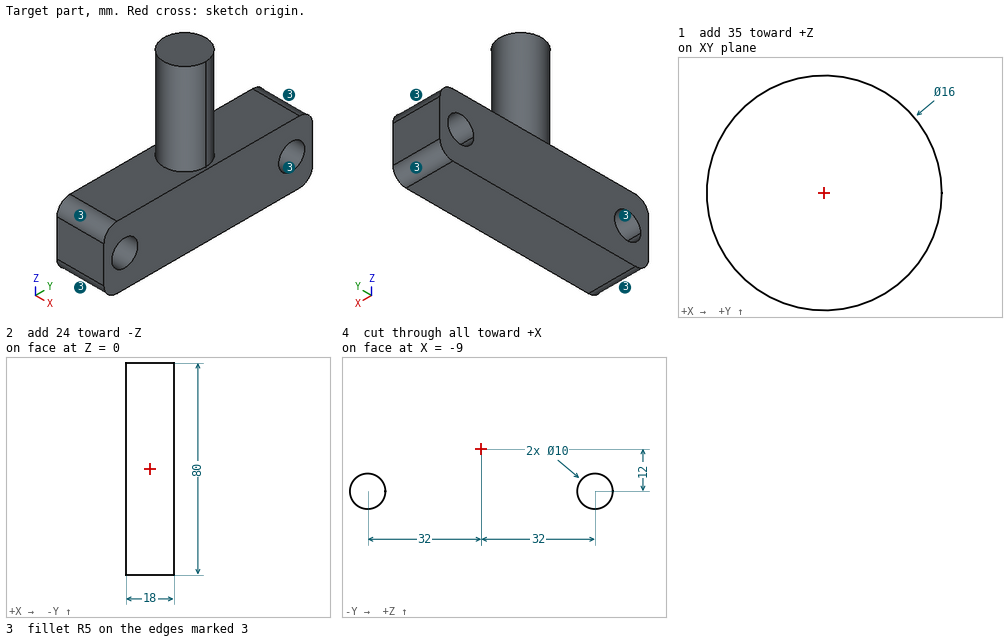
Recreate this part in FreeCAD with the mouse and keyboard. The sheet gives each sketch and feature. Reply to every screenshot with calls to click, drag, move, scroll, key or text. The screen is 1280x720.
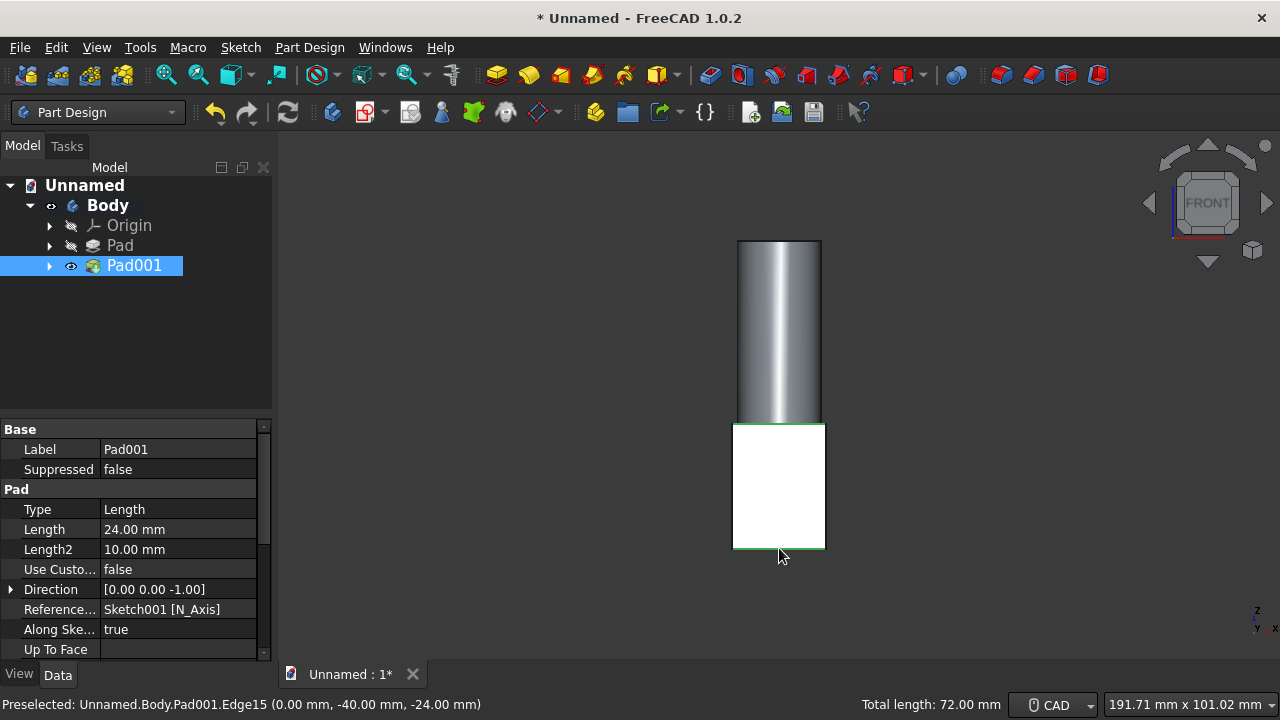
click(1002, 76)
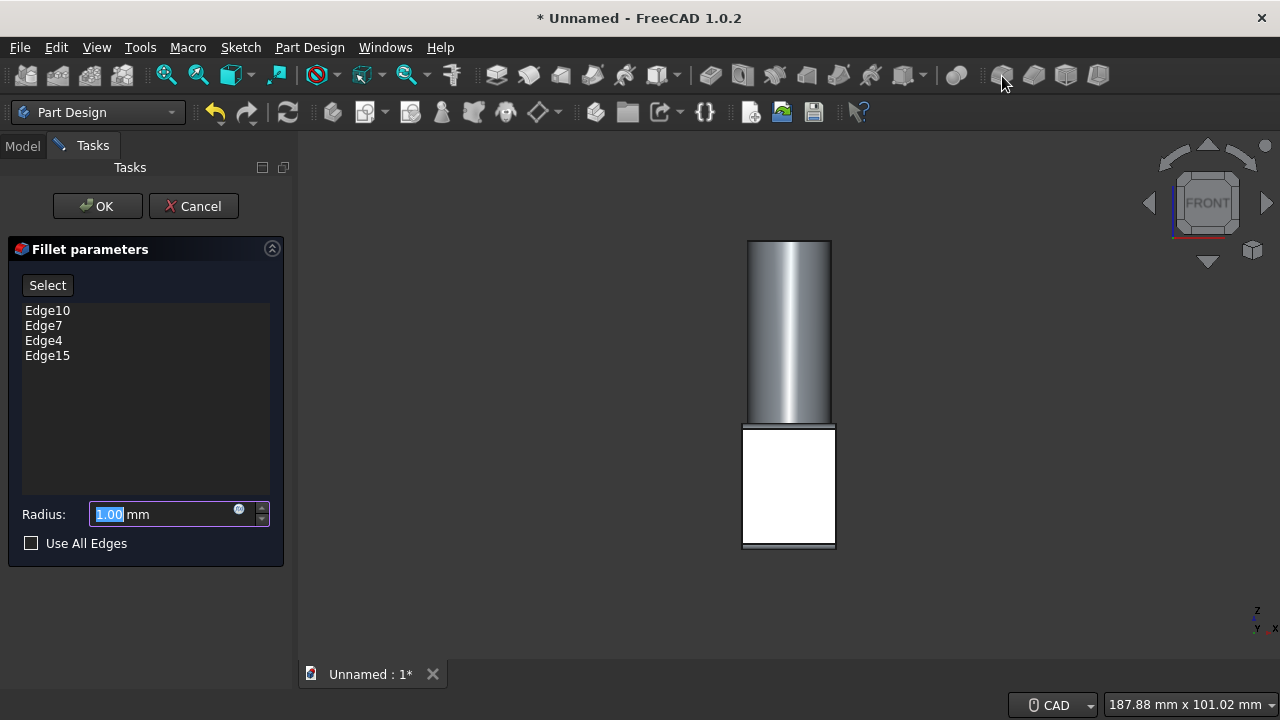
text(5)
key(Tab)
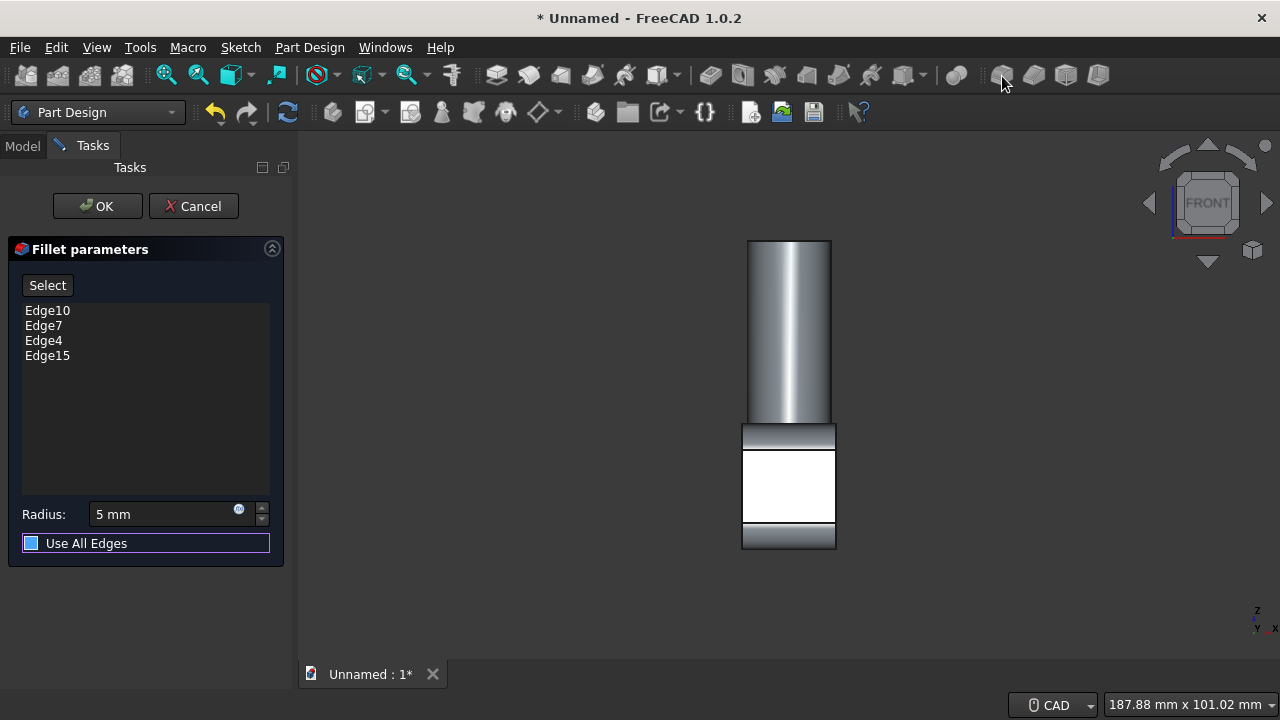
click(98, 206)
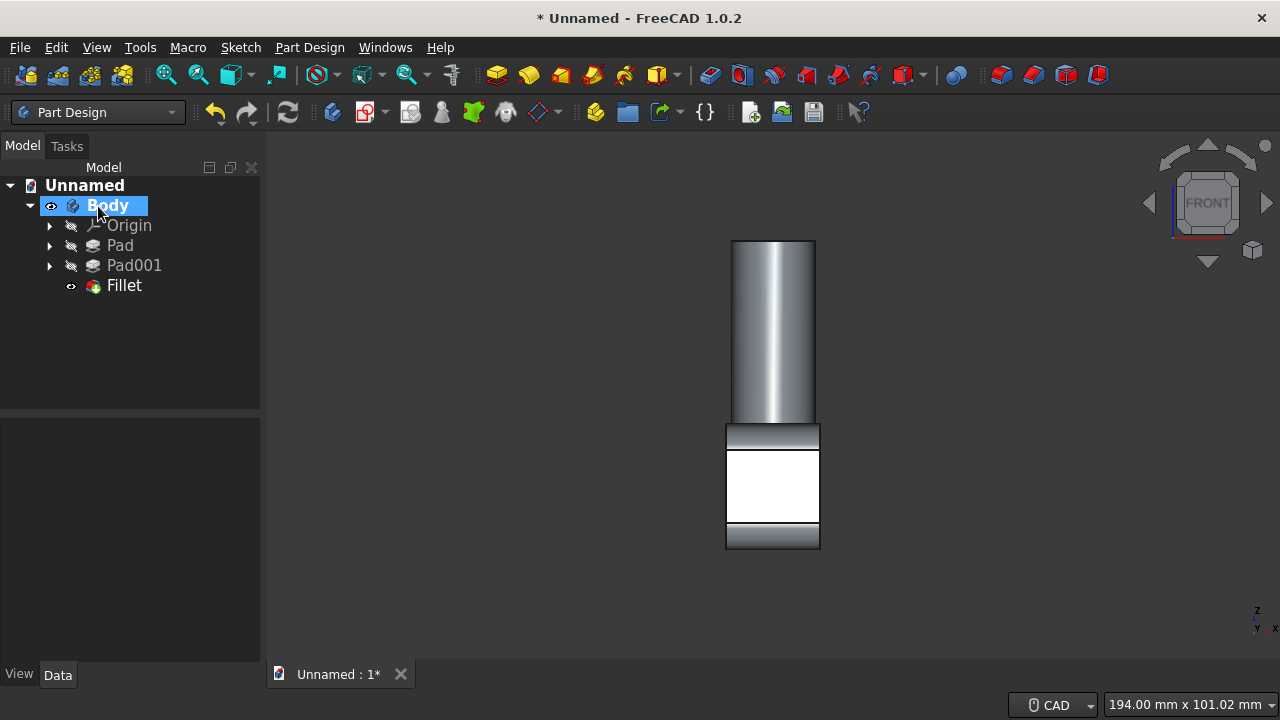
key(6)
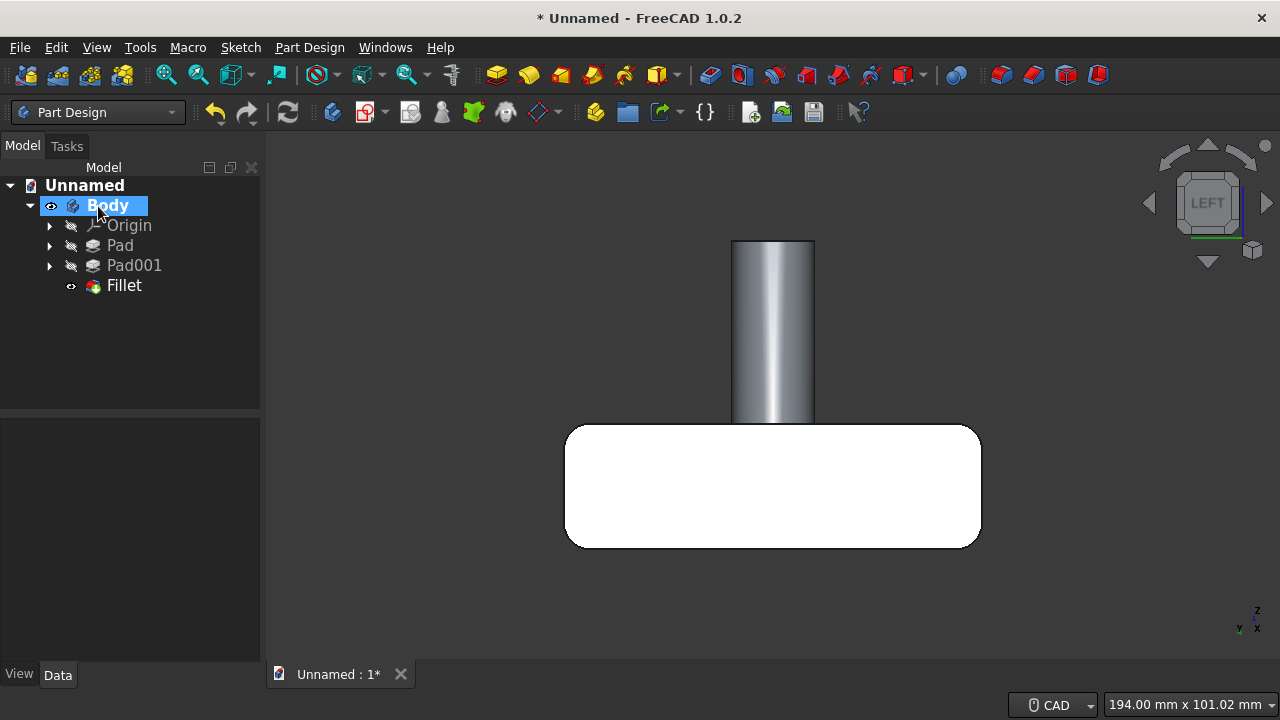
click(654, 485)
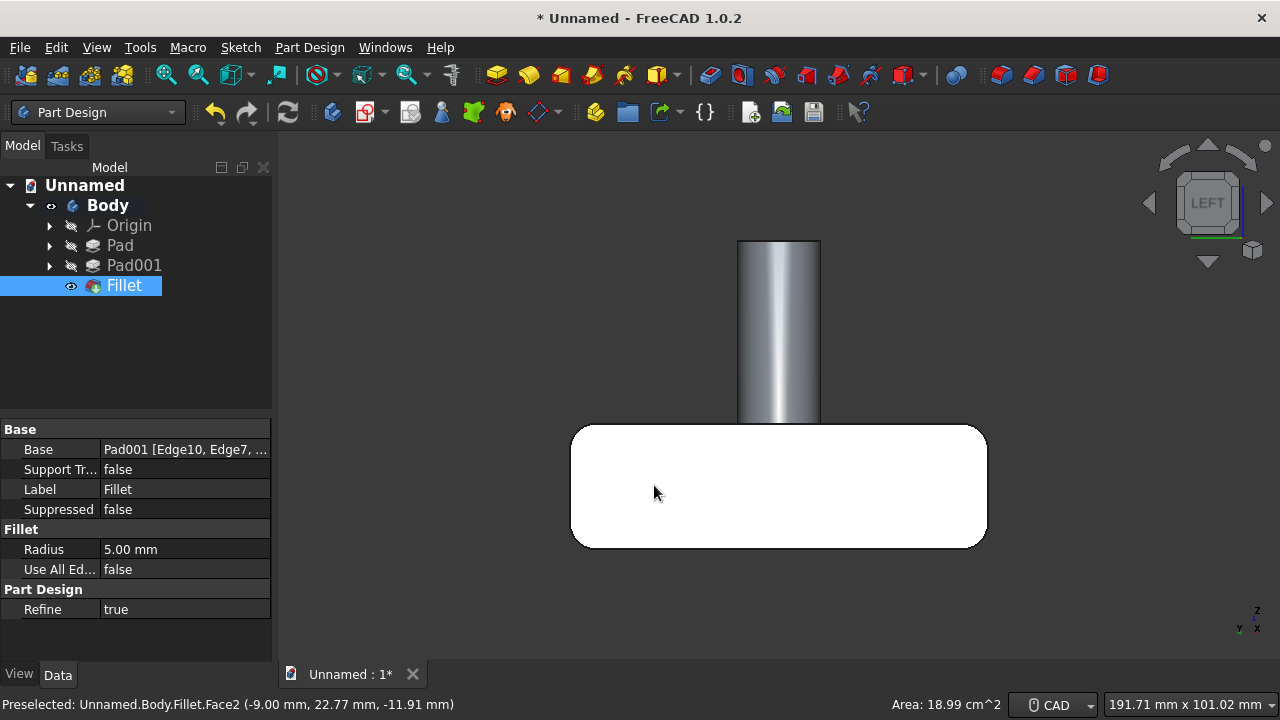
click(366, 112)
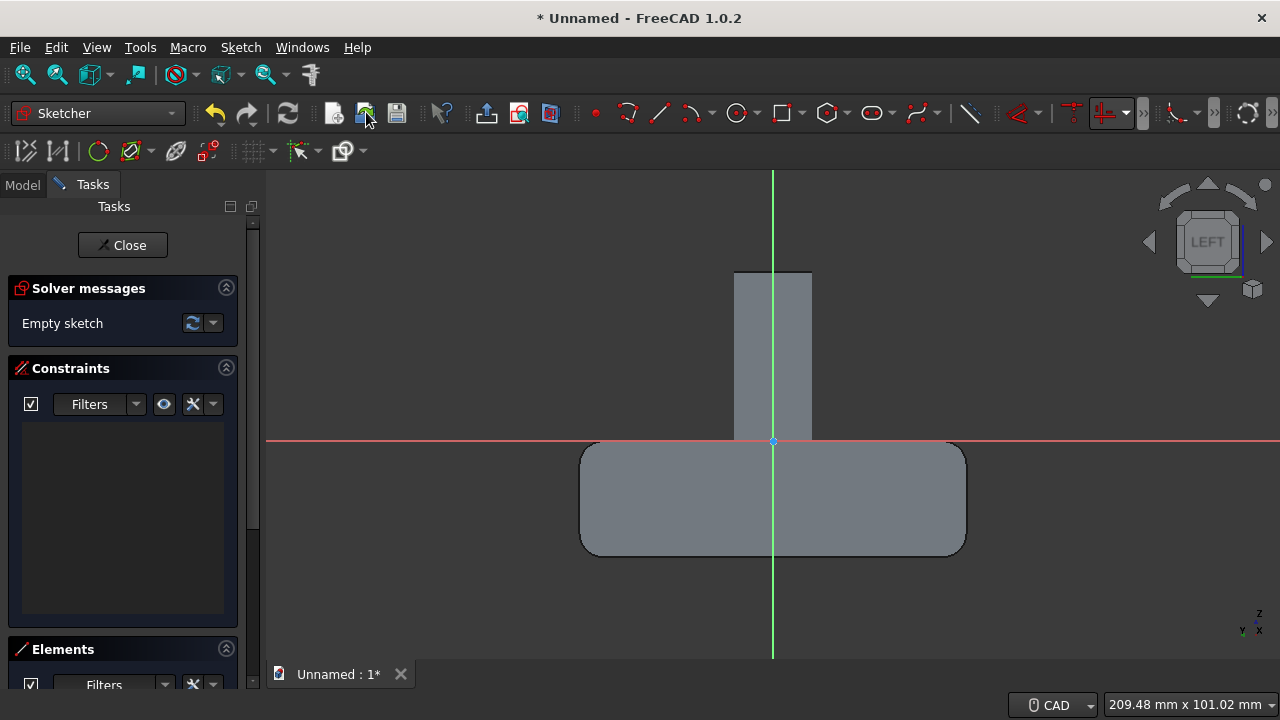
scroll(912, 620, up, 2)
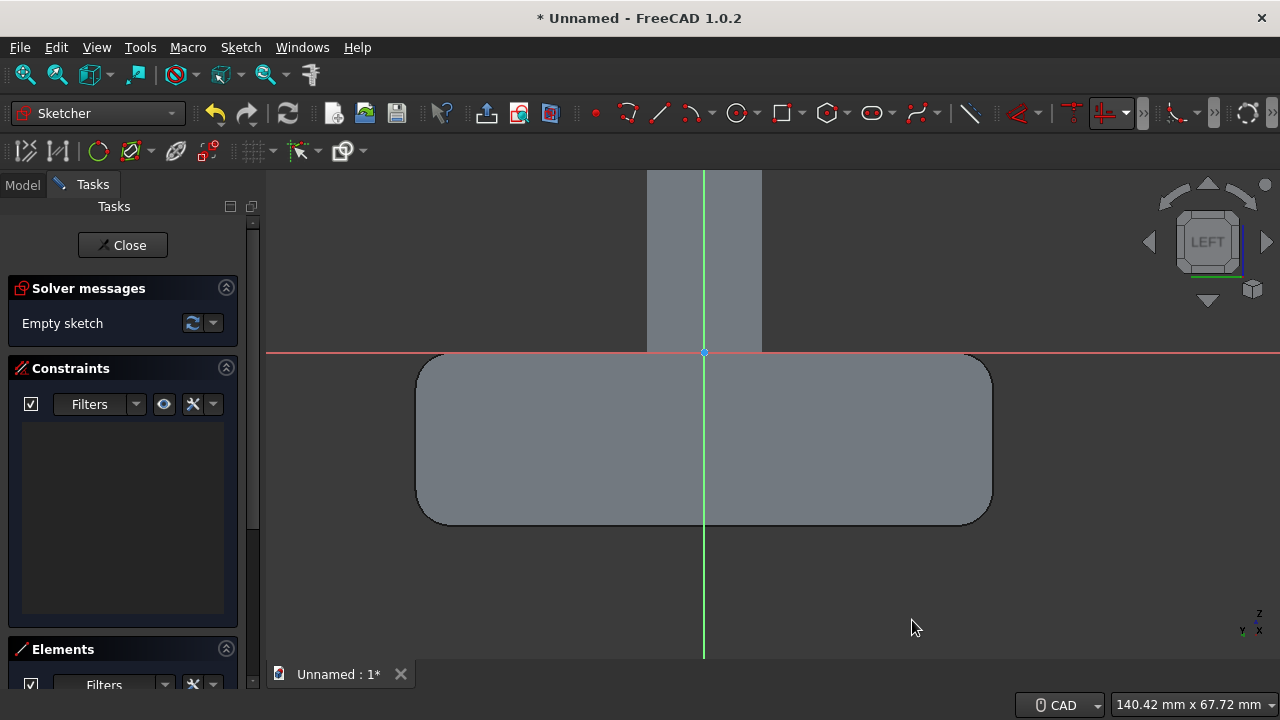
click(738, 114)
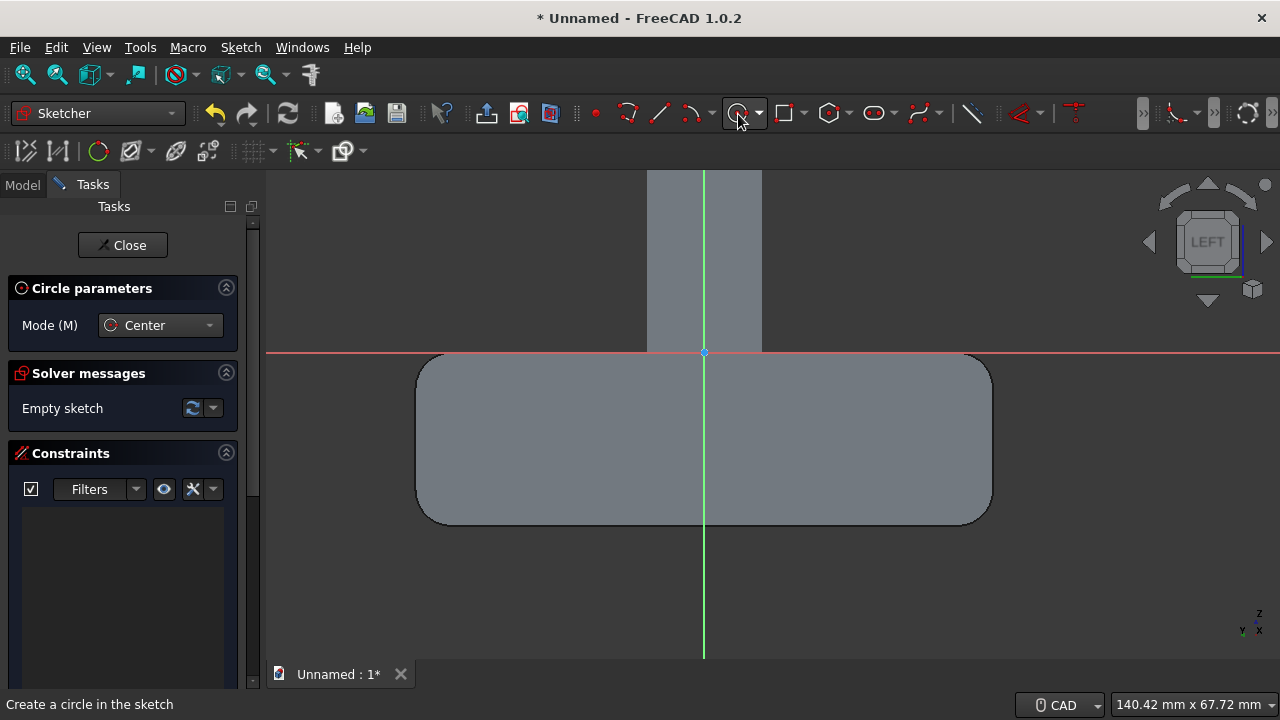
click(935, 439)
move(961, 414)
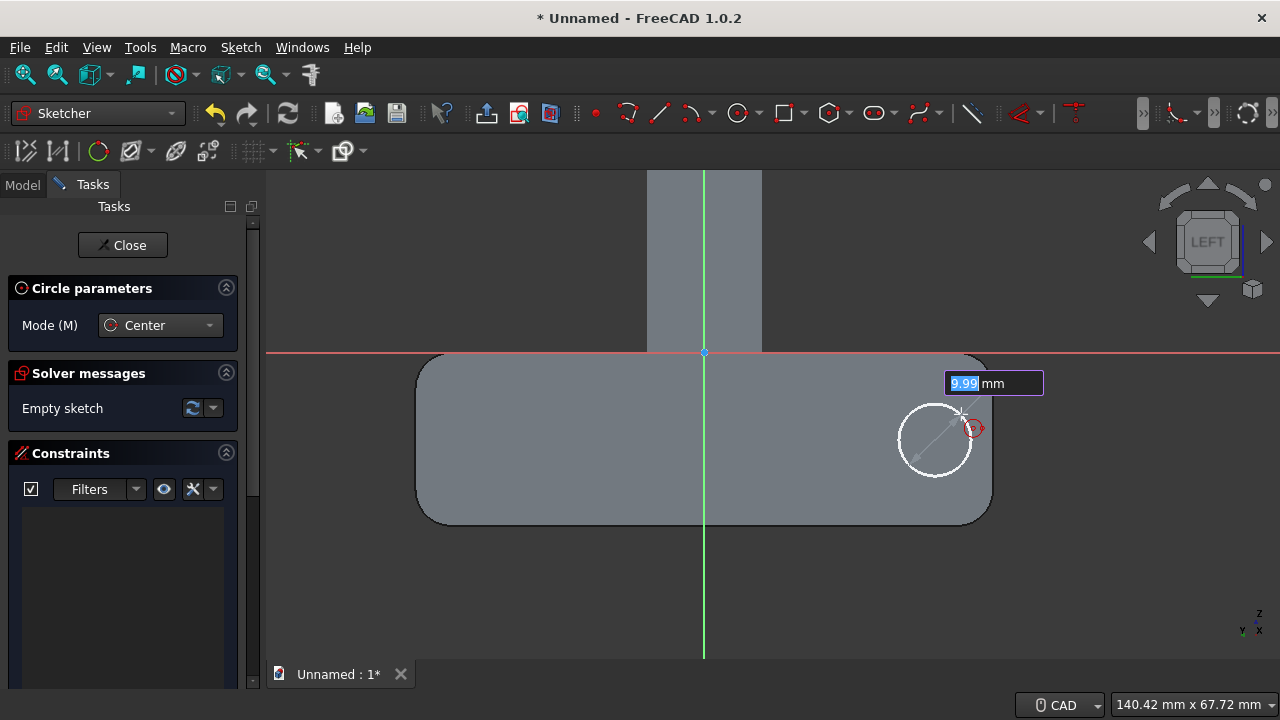
text(10)
key(Return)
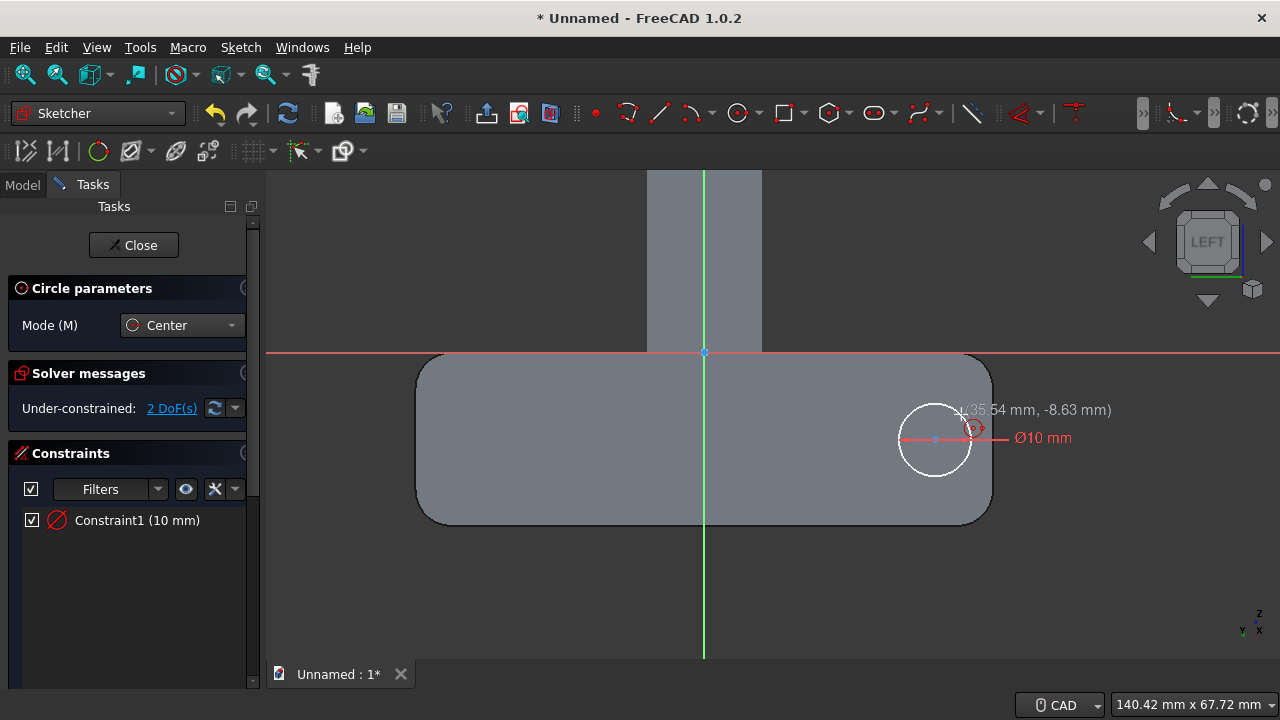
click(473, 439)
move(499, 414)